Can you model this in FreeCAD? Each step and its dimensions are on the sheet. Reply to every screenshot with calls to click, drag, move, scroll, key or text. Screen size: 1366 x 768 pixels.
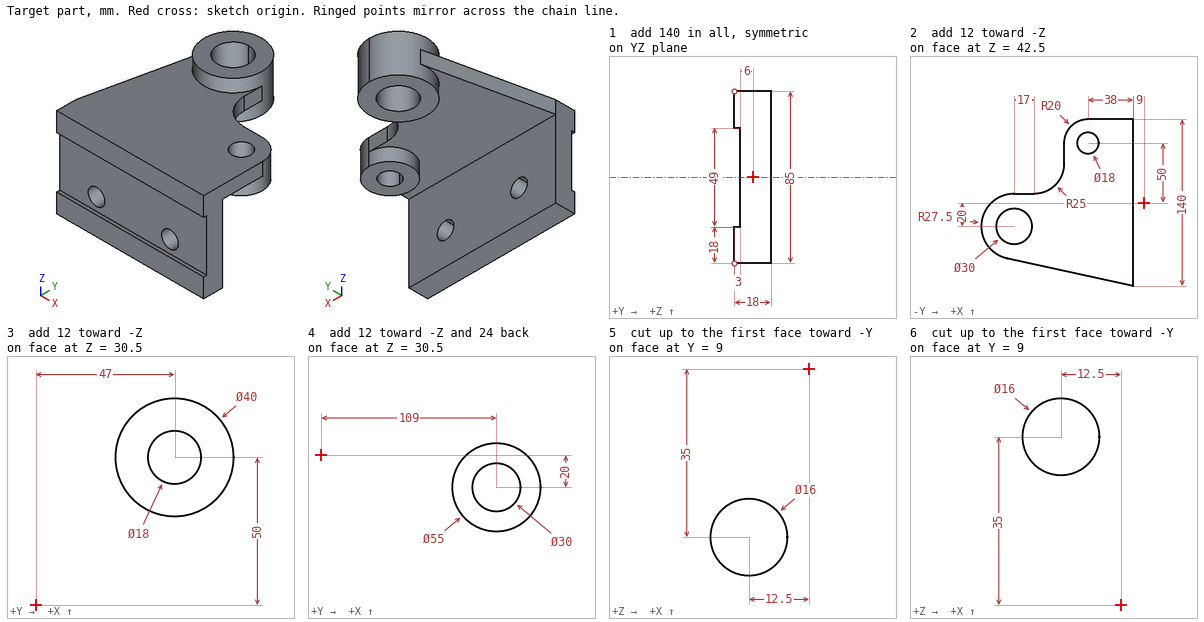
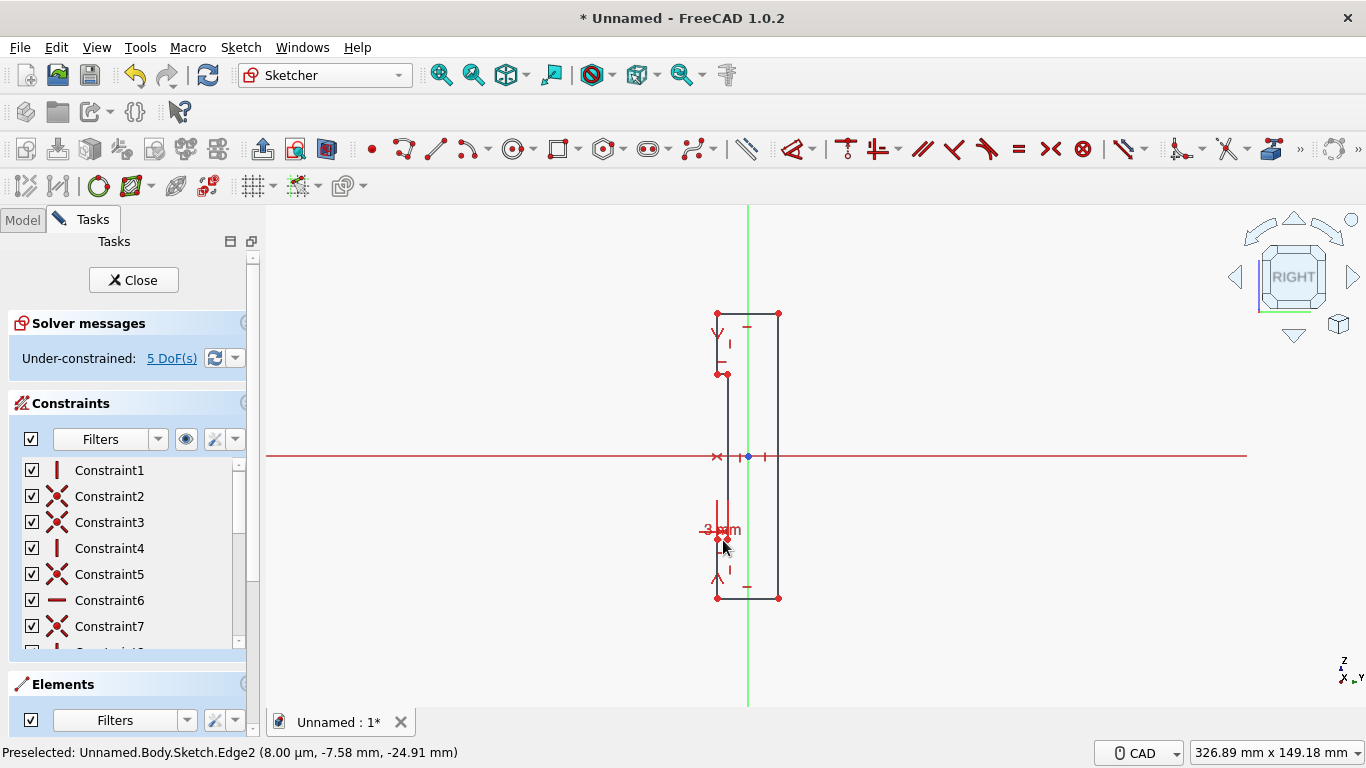
click(728, 490)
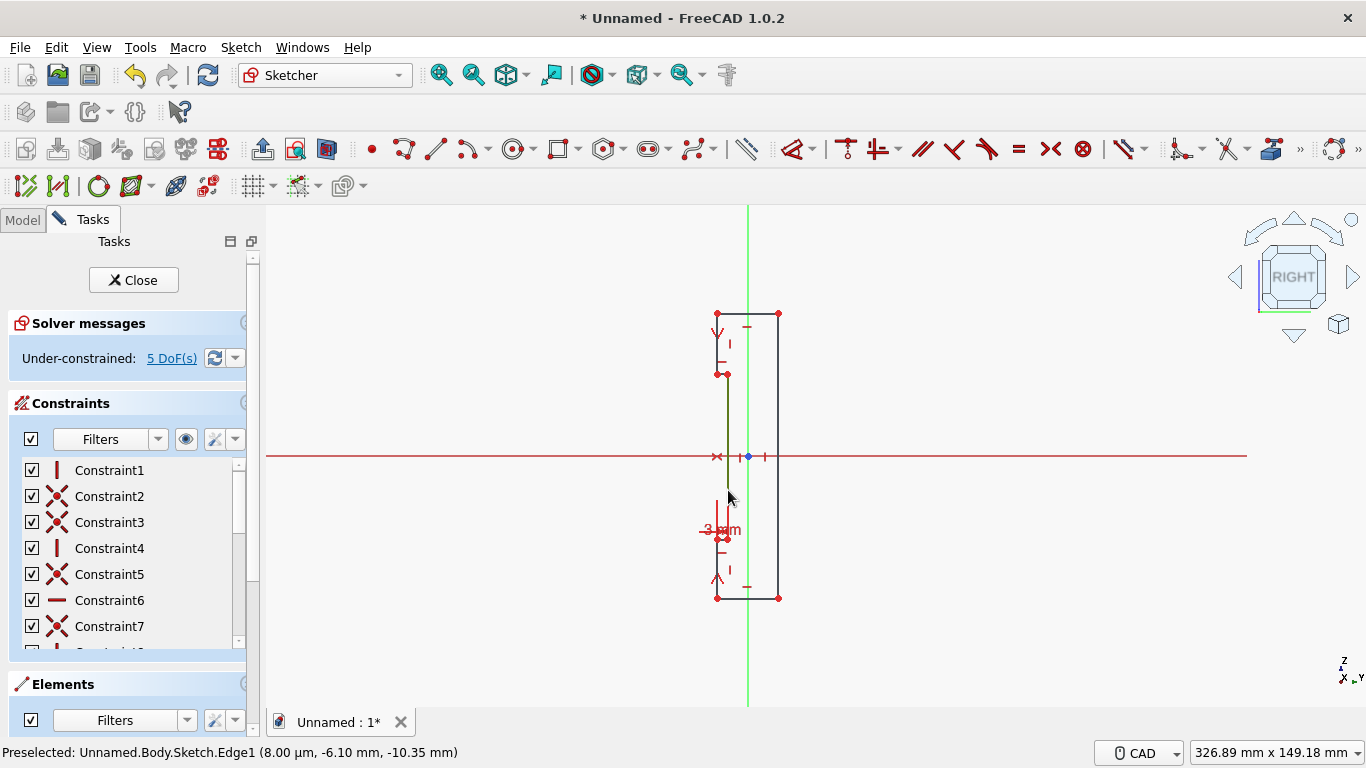
click(814, 150)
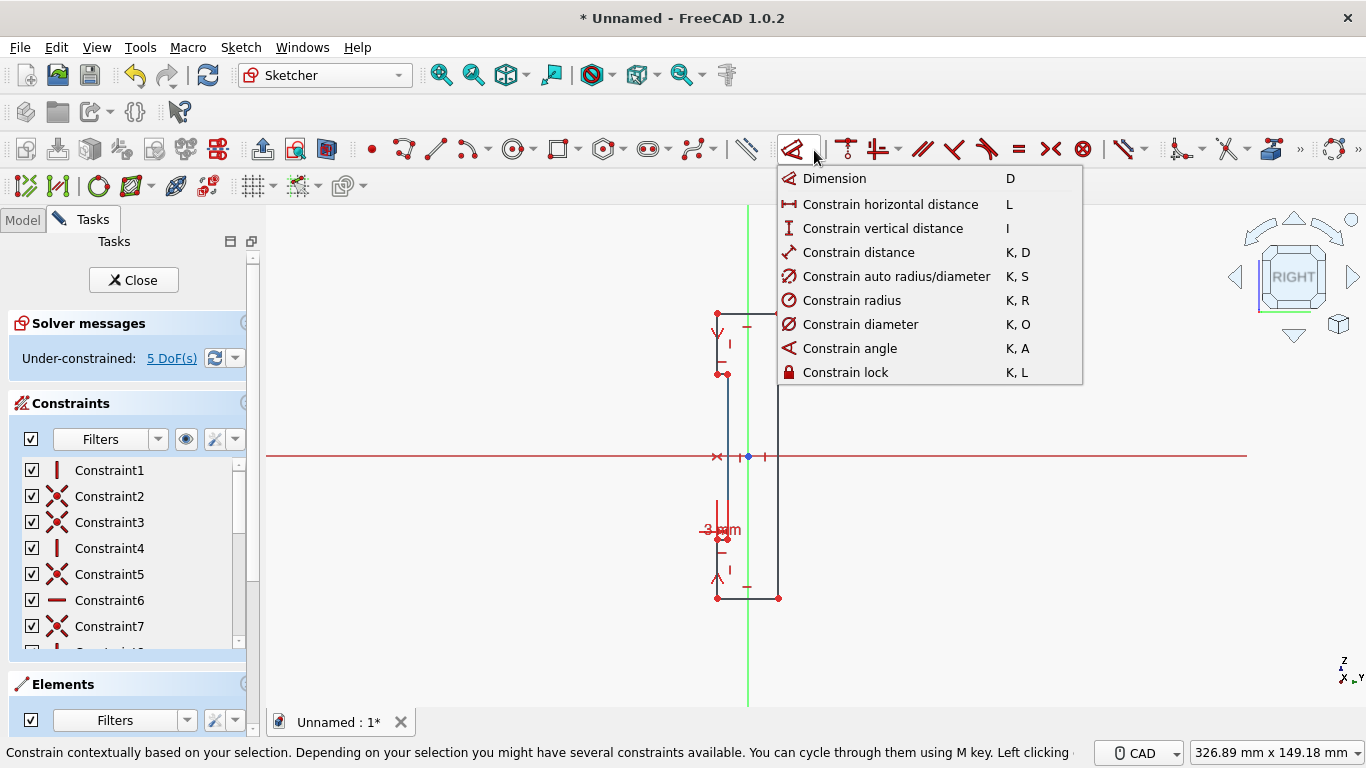
click(930, 228)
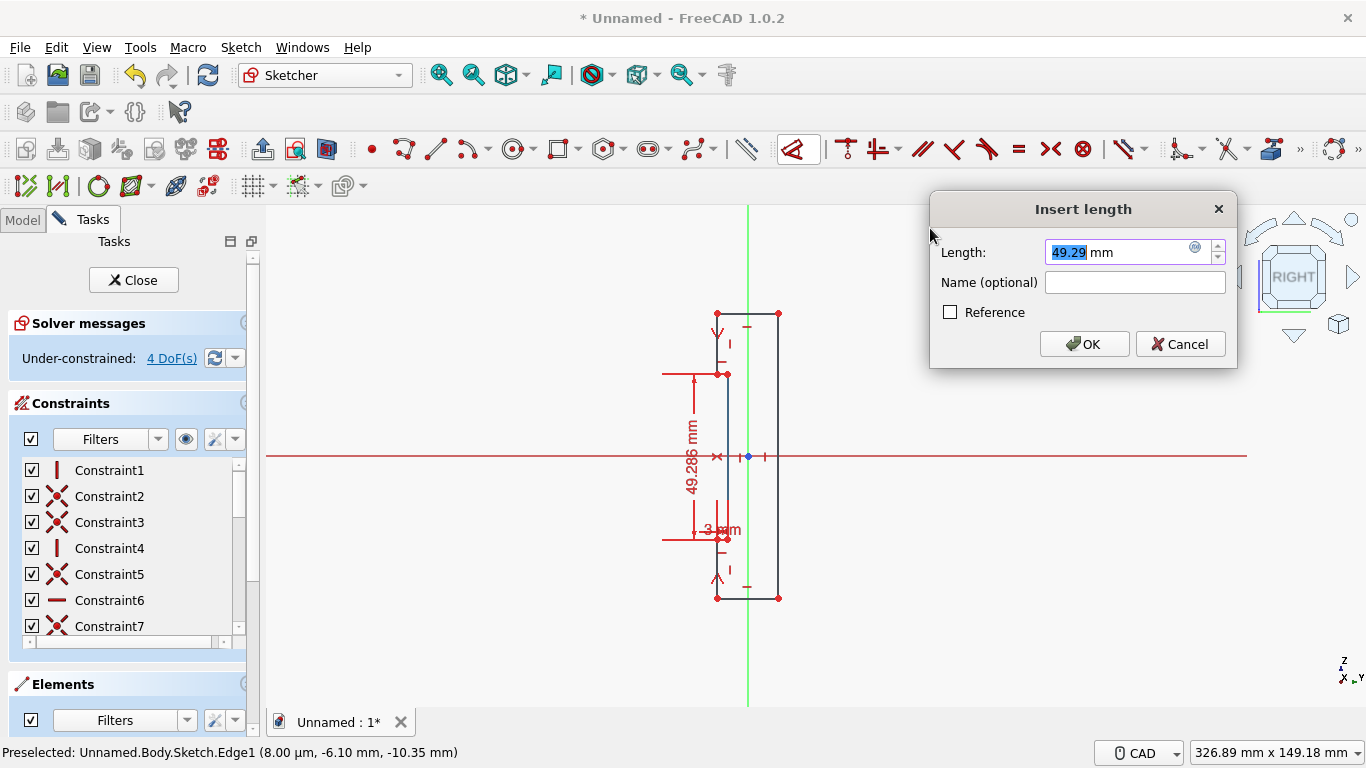
text(49)
key(Return)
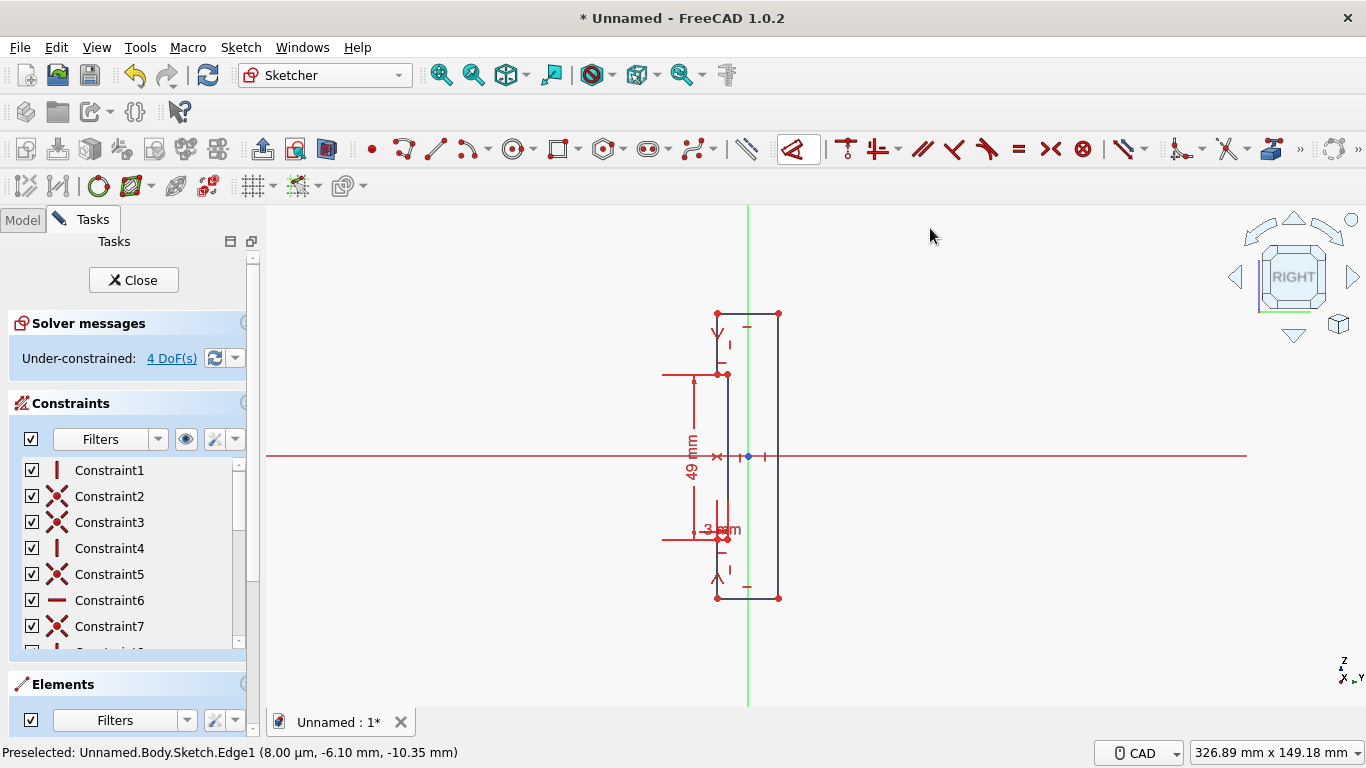
click(717, 581)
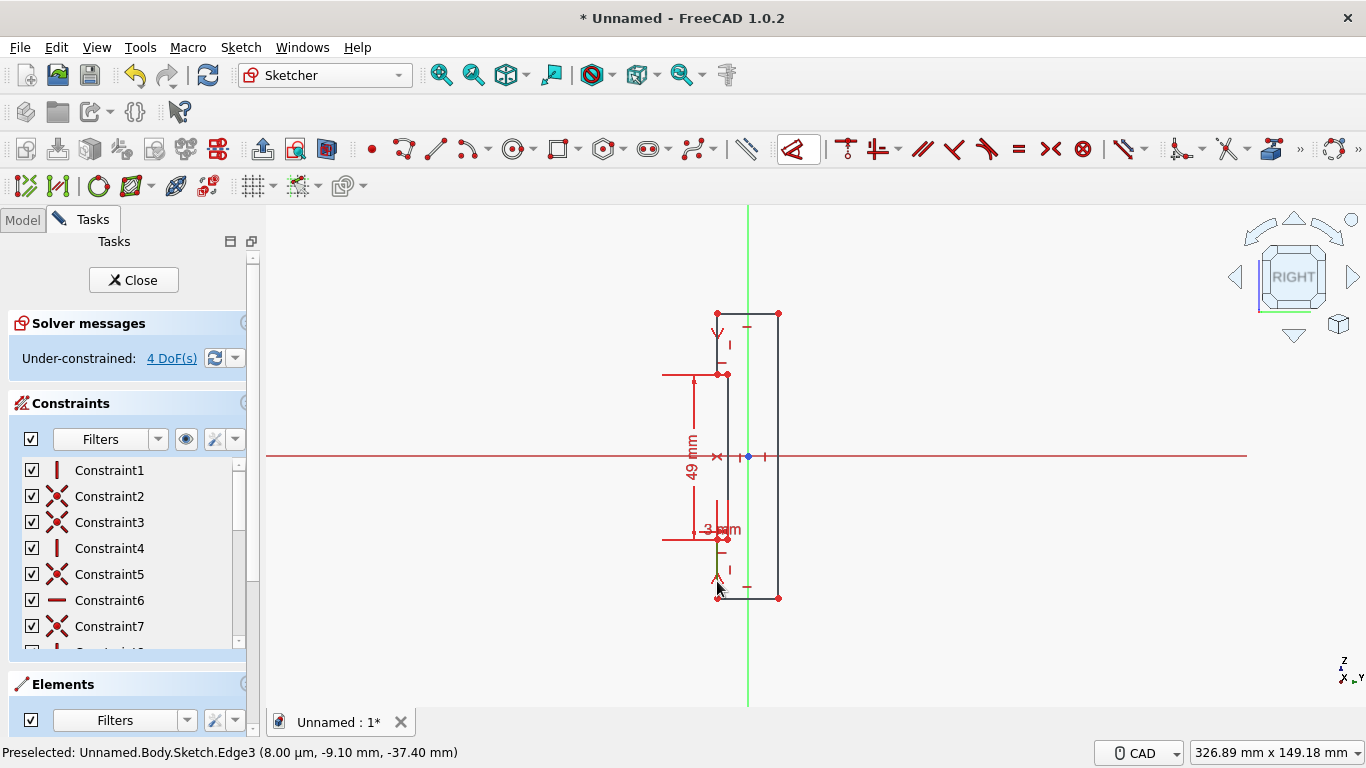
key(i)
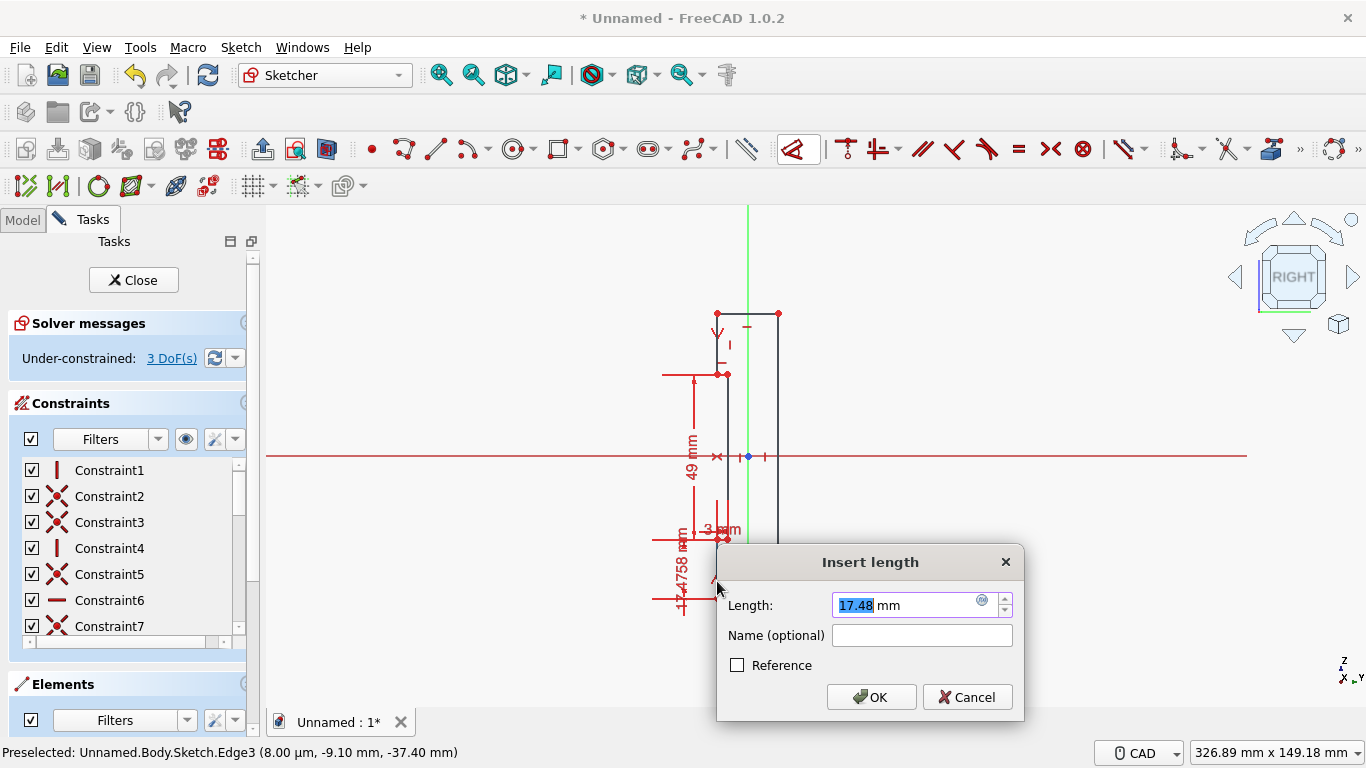
text(18)
key(Return)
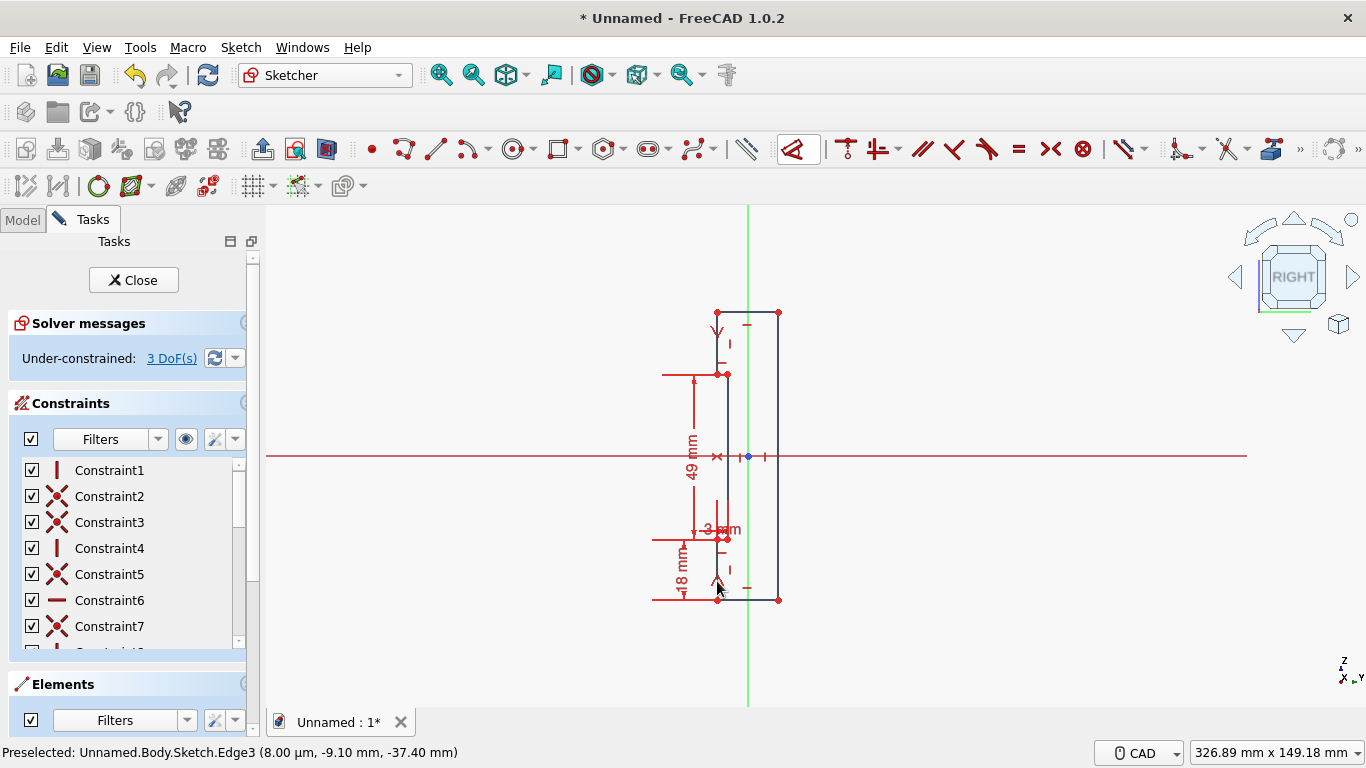
click(736, 600)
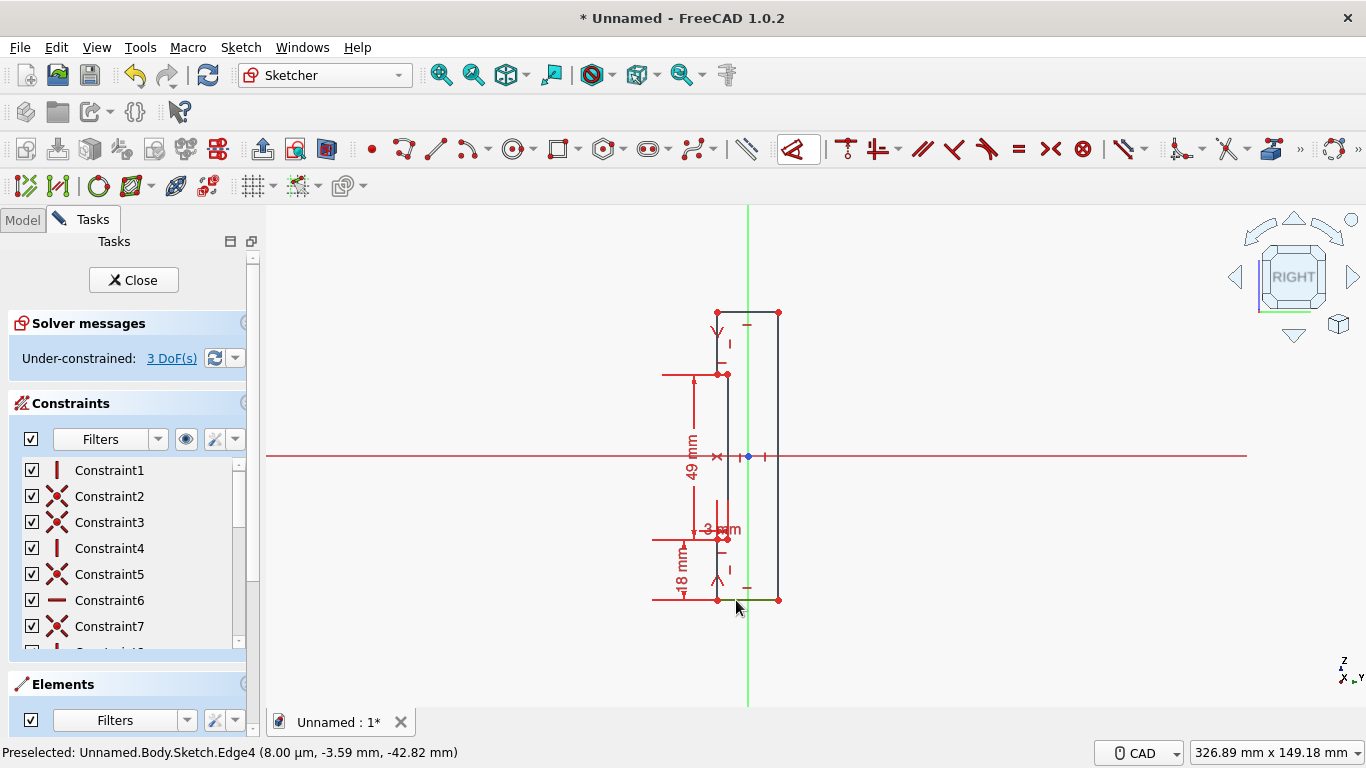
key(l)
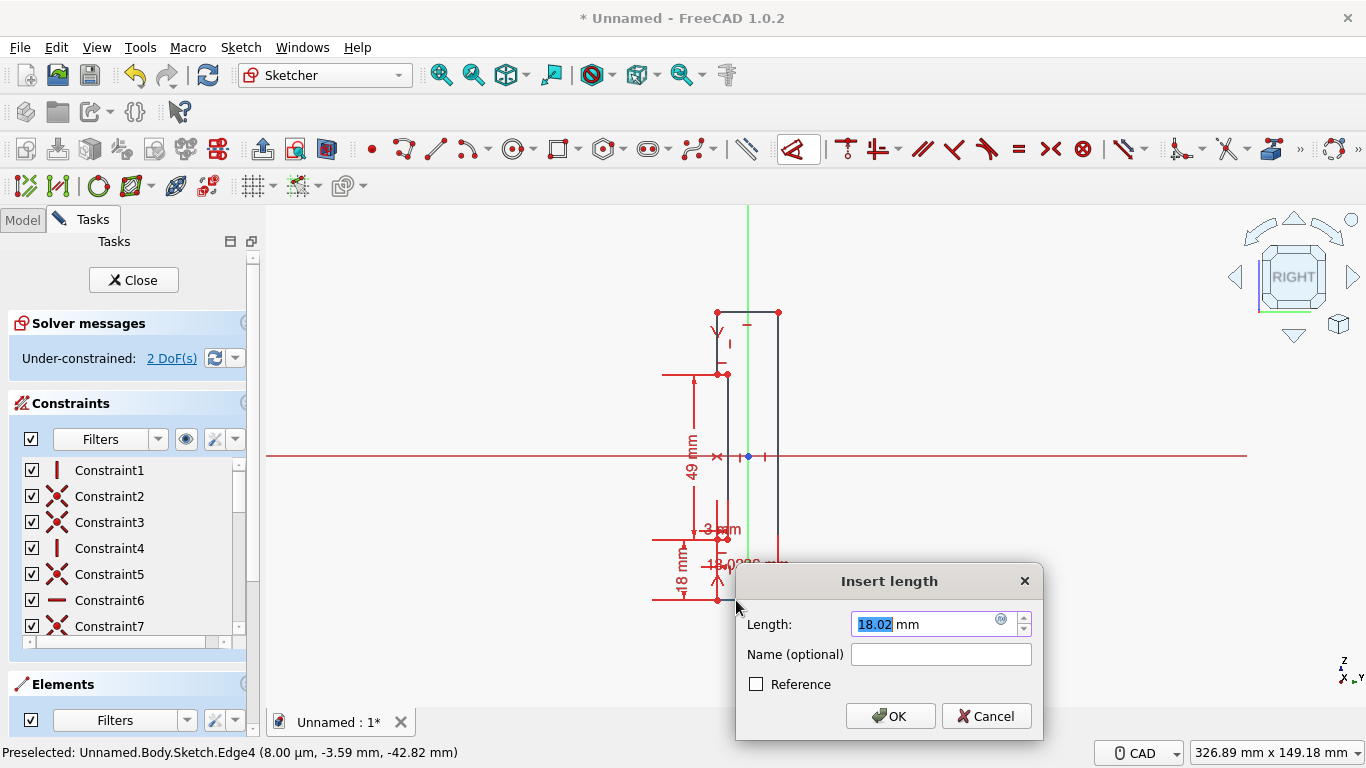
text(18)
key(Return)